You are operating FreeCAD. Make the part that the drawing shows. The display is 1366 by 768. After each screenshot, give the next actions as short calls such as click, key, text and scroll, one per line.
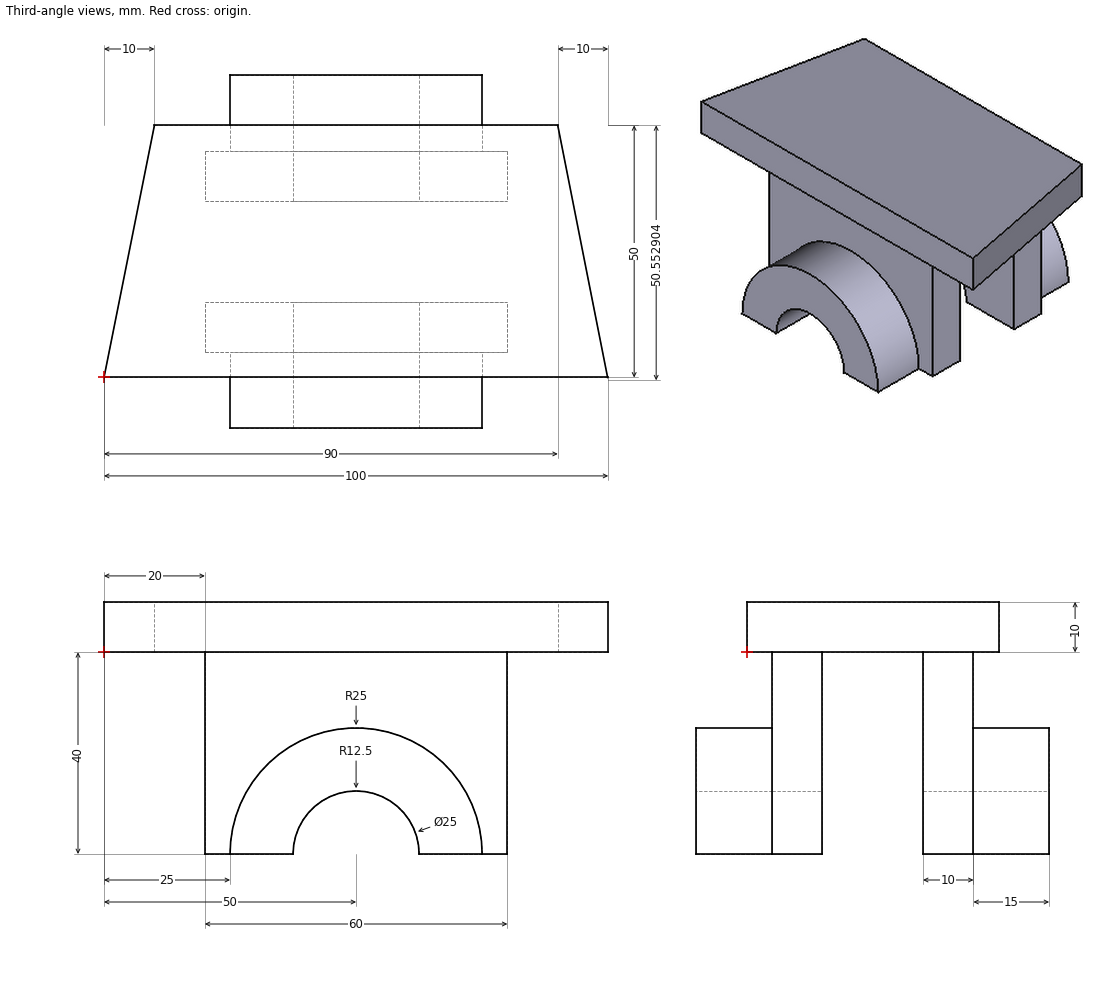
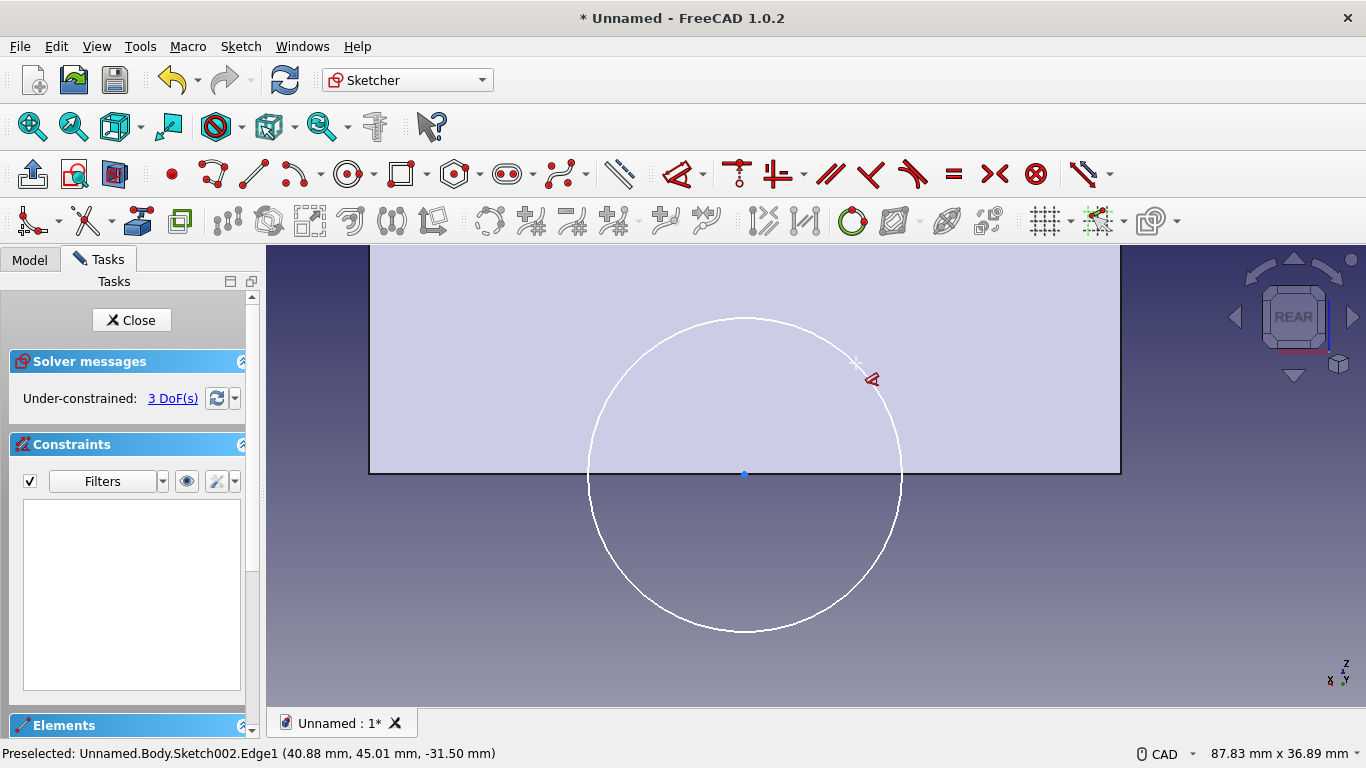
click(856, 364)
click(879, 341)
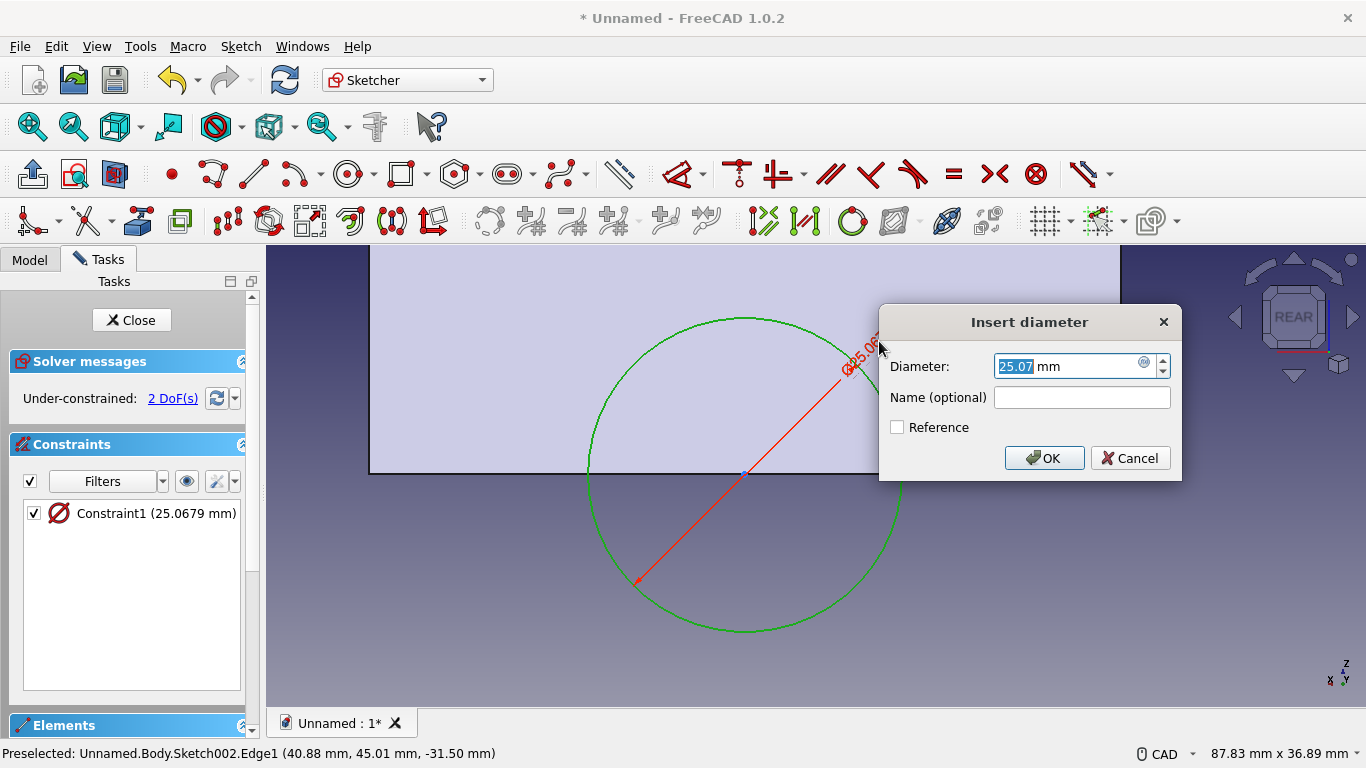
text(25)
key(Return)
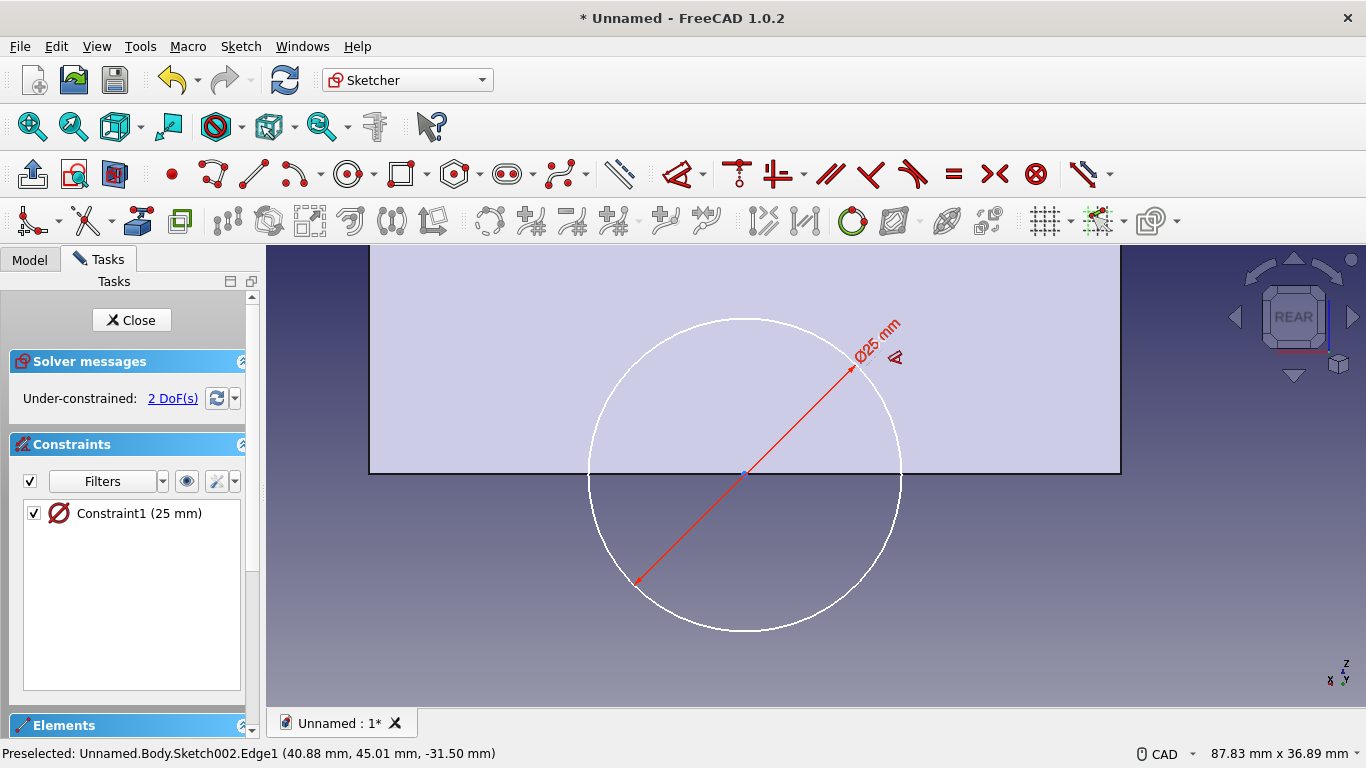
click(745, 475)
click(973, 509)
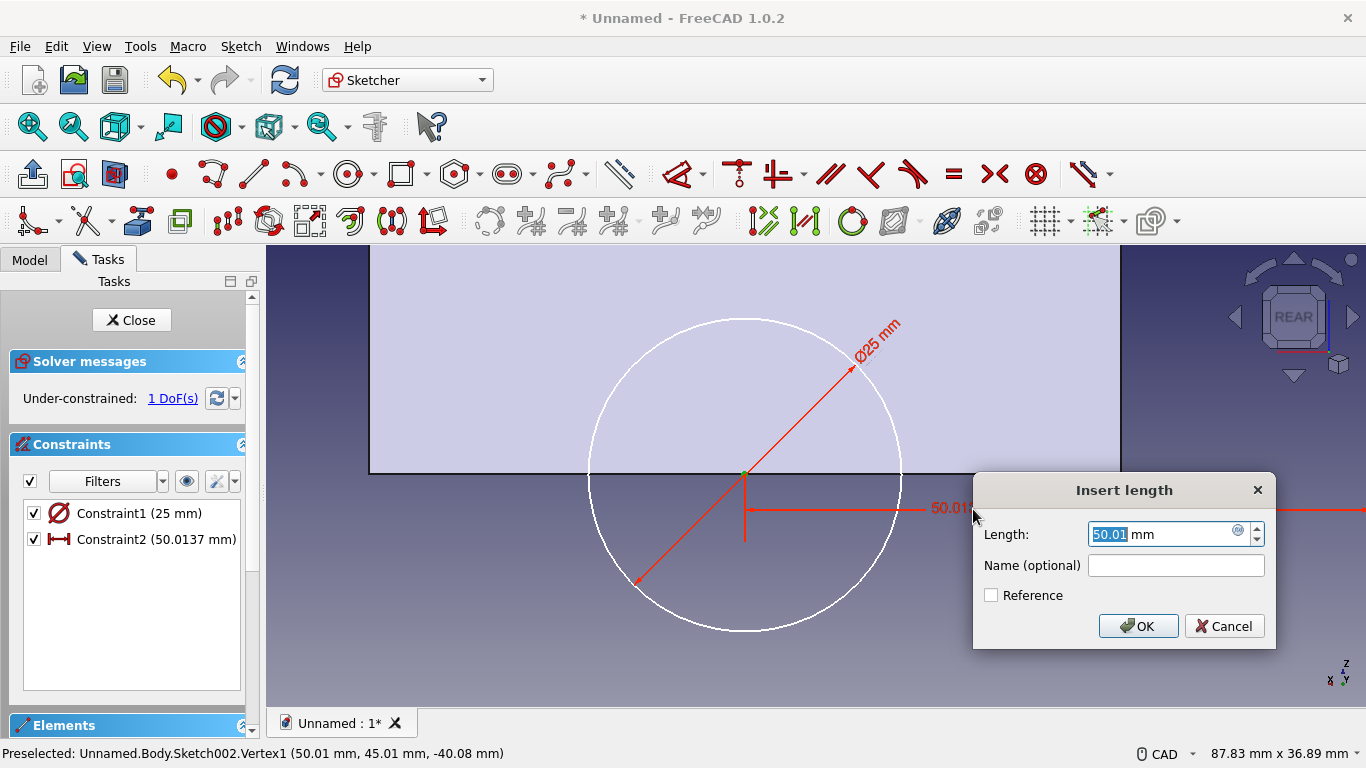
text(50)
key(Return)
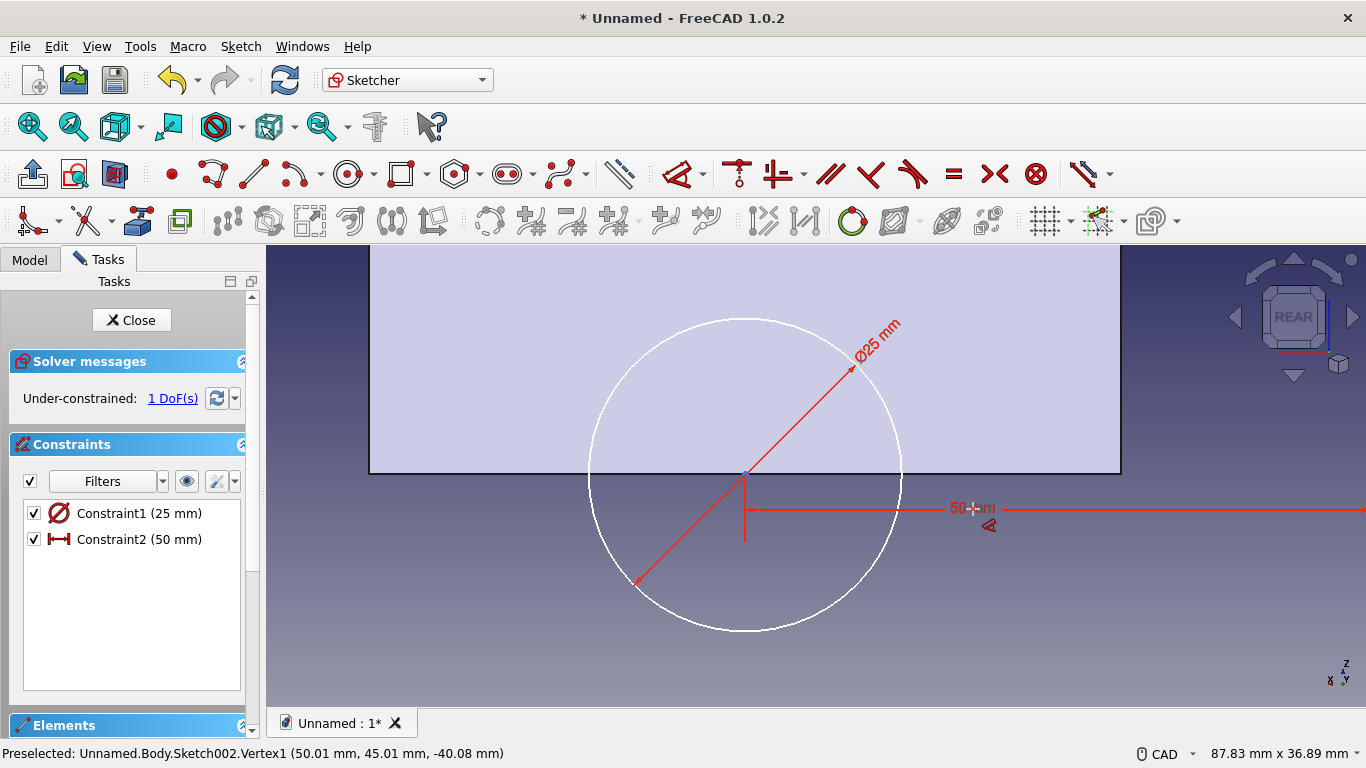
click(745, 475)
click(711, 374)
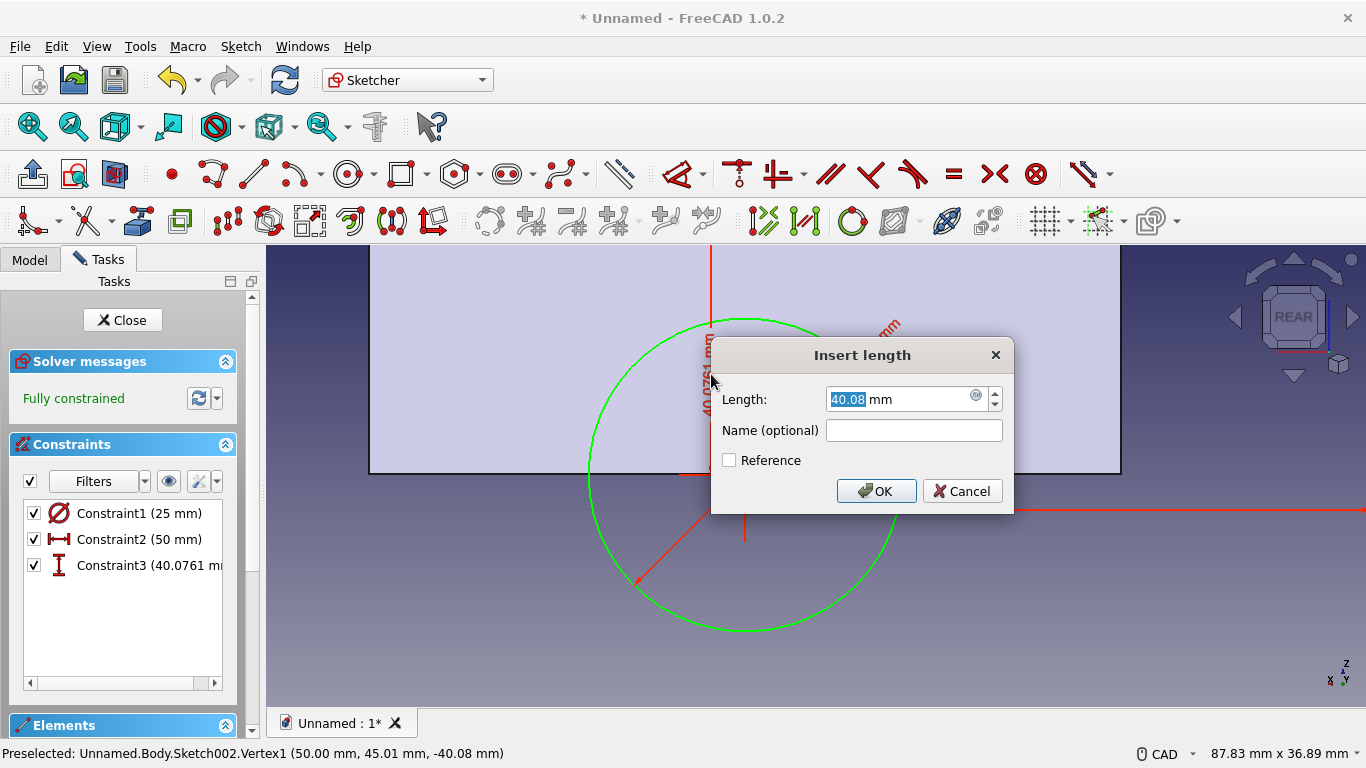
text(40)
key(Return)
key(Escape)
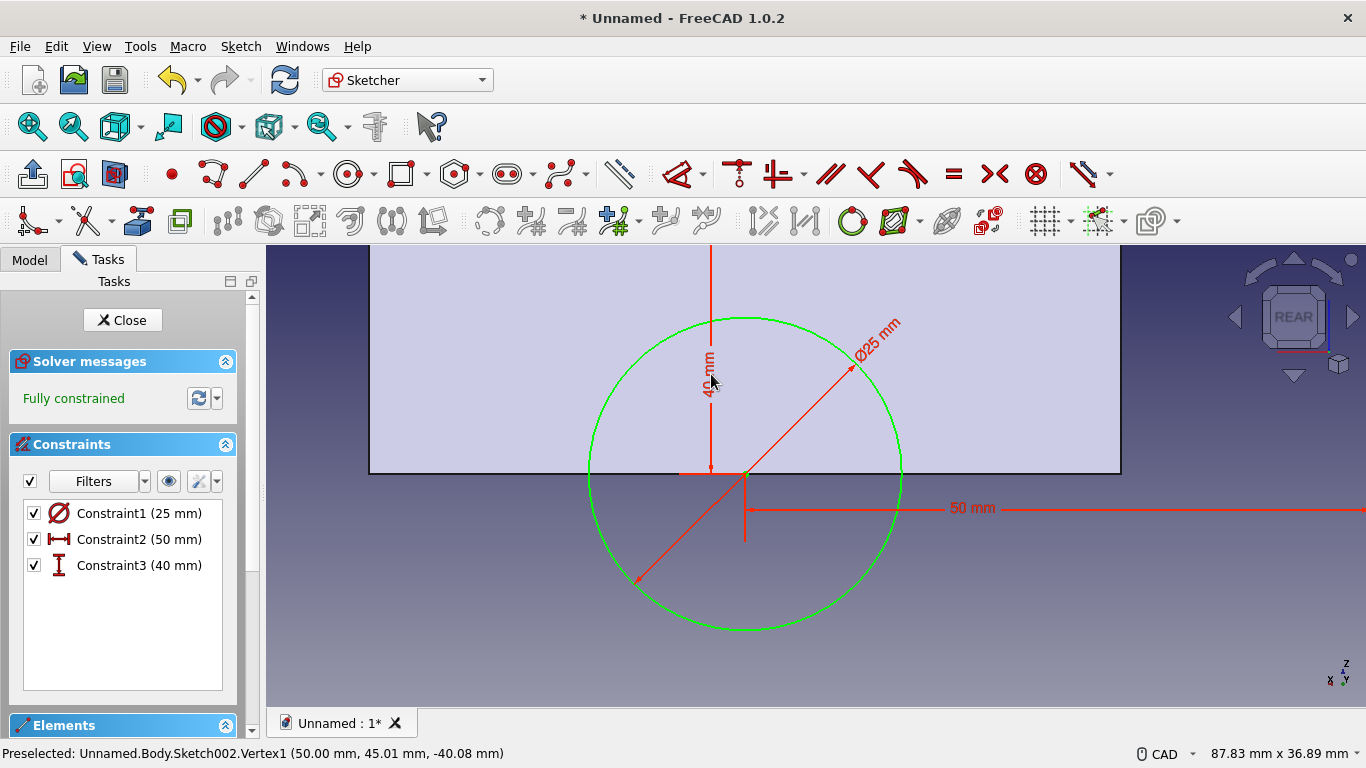
click(123, 320)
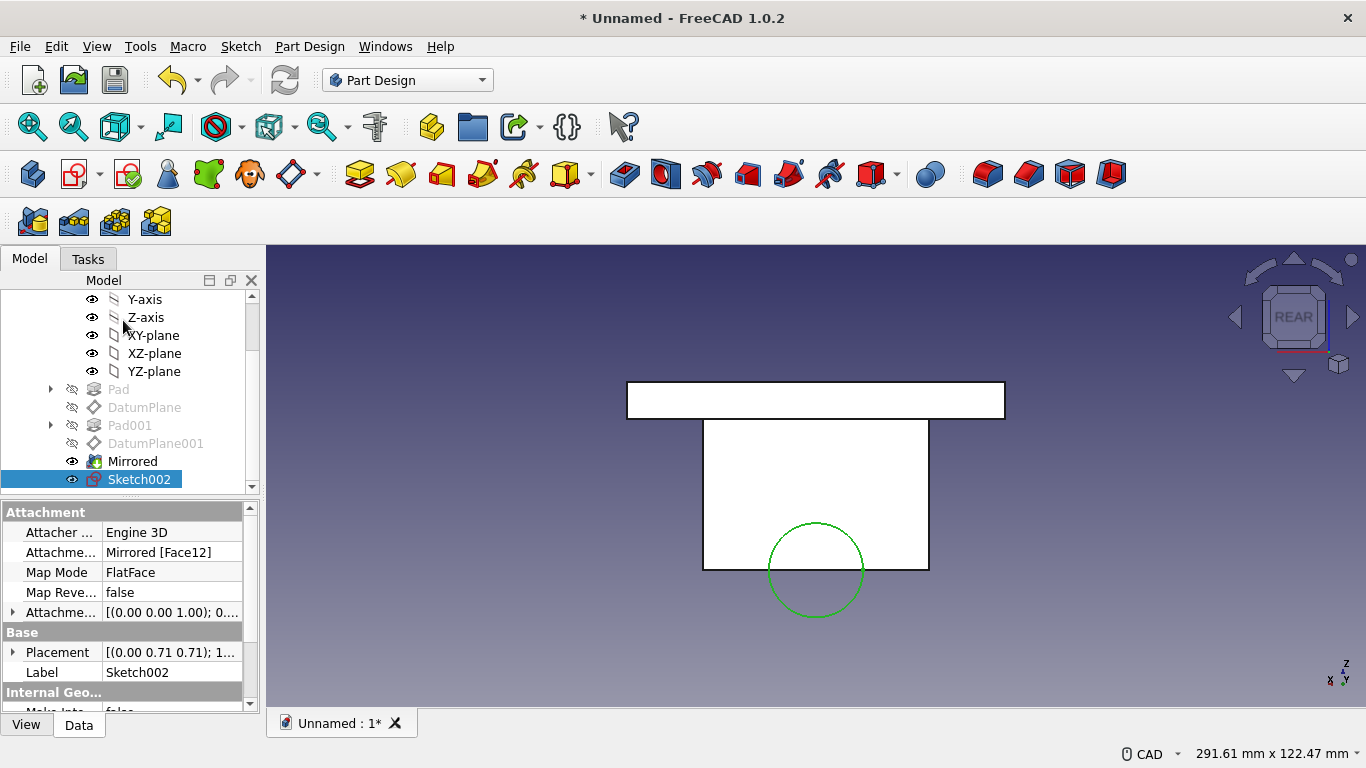
click(625, 174)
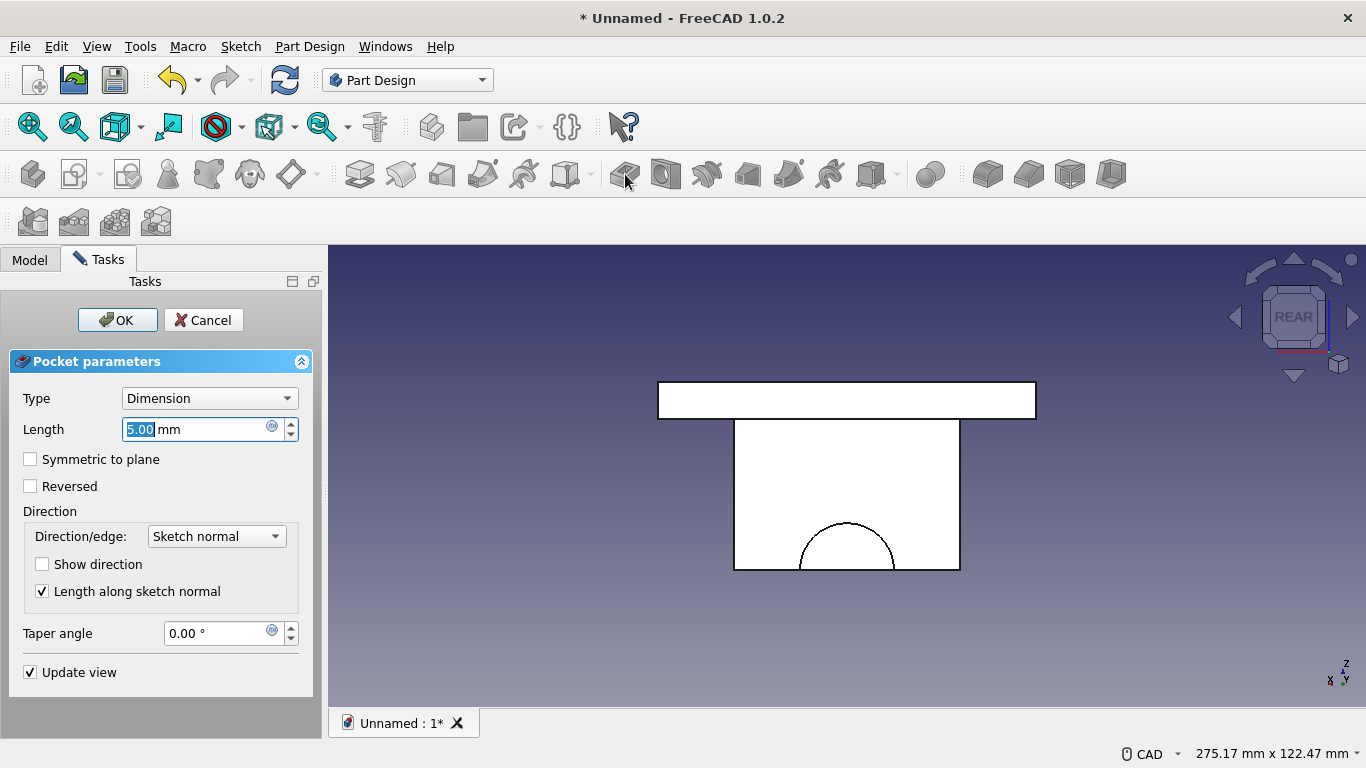
click(210, 398)